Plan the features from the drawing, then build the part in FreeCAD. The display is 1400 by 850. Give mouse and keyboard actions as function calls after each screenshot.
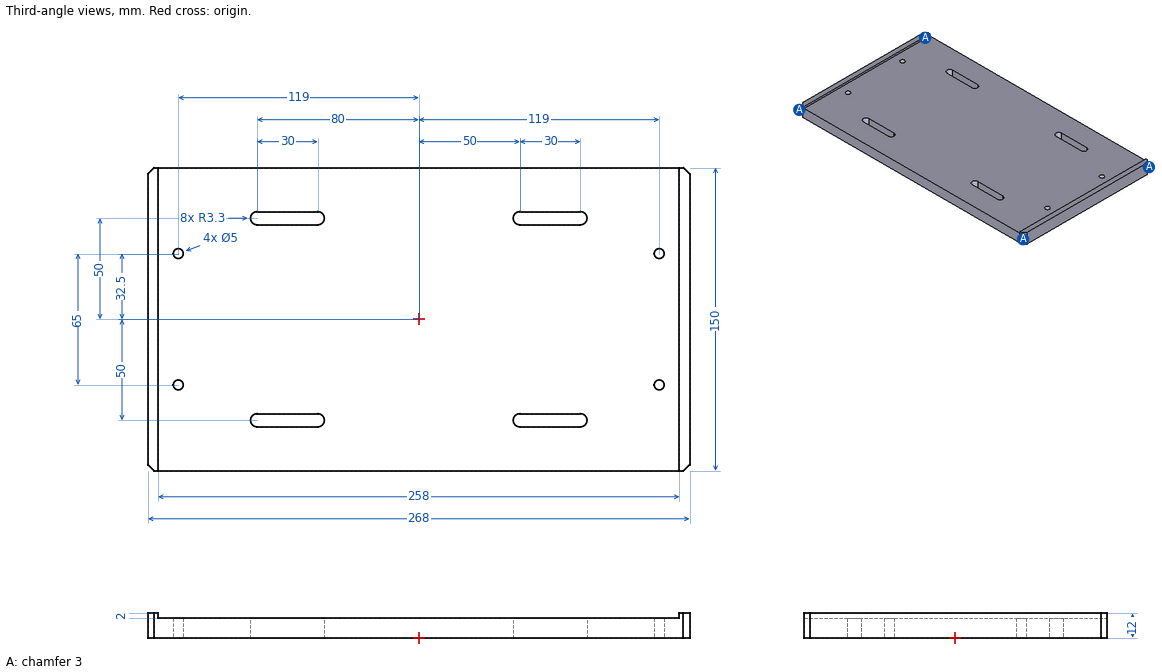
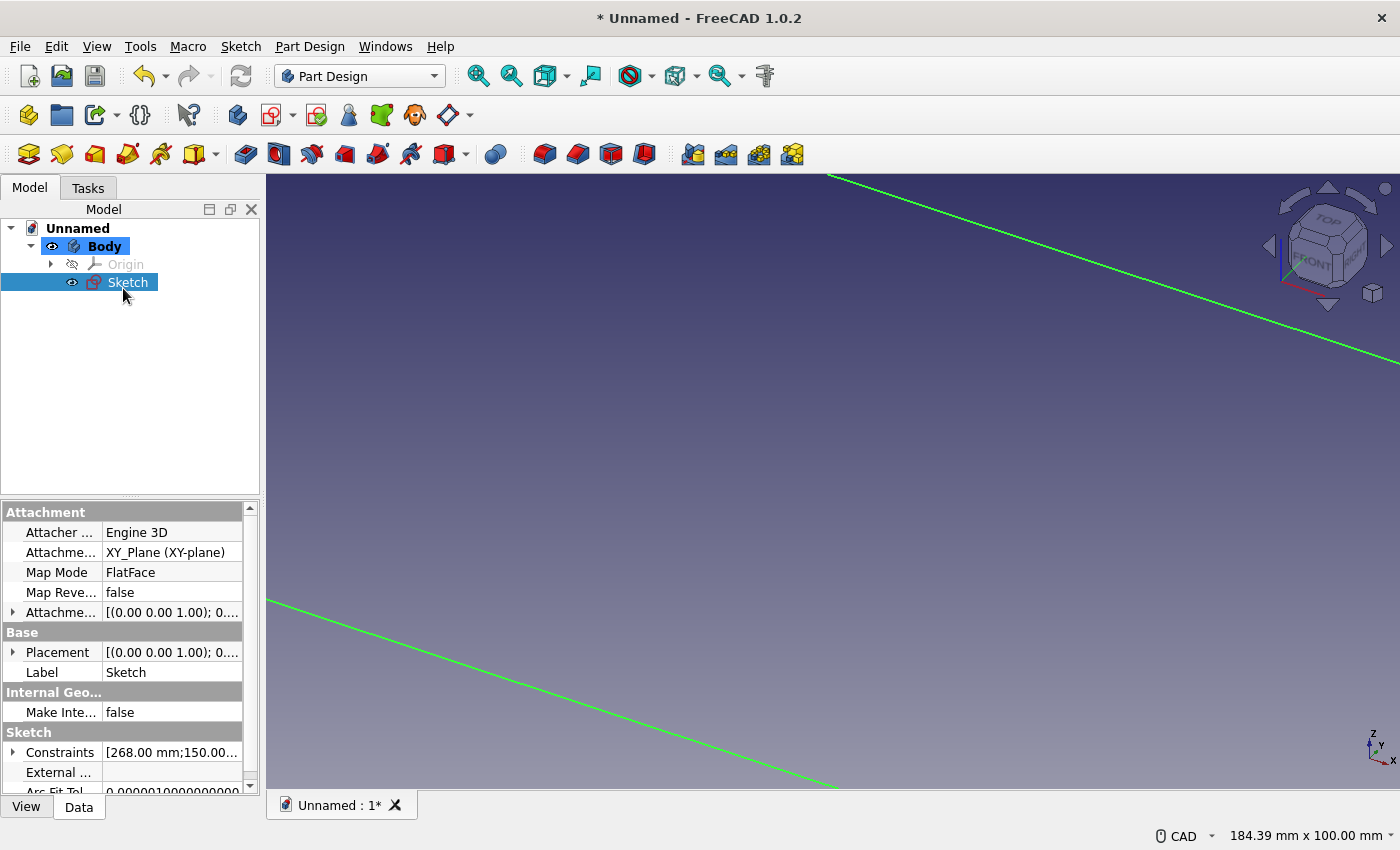
click(29, 154)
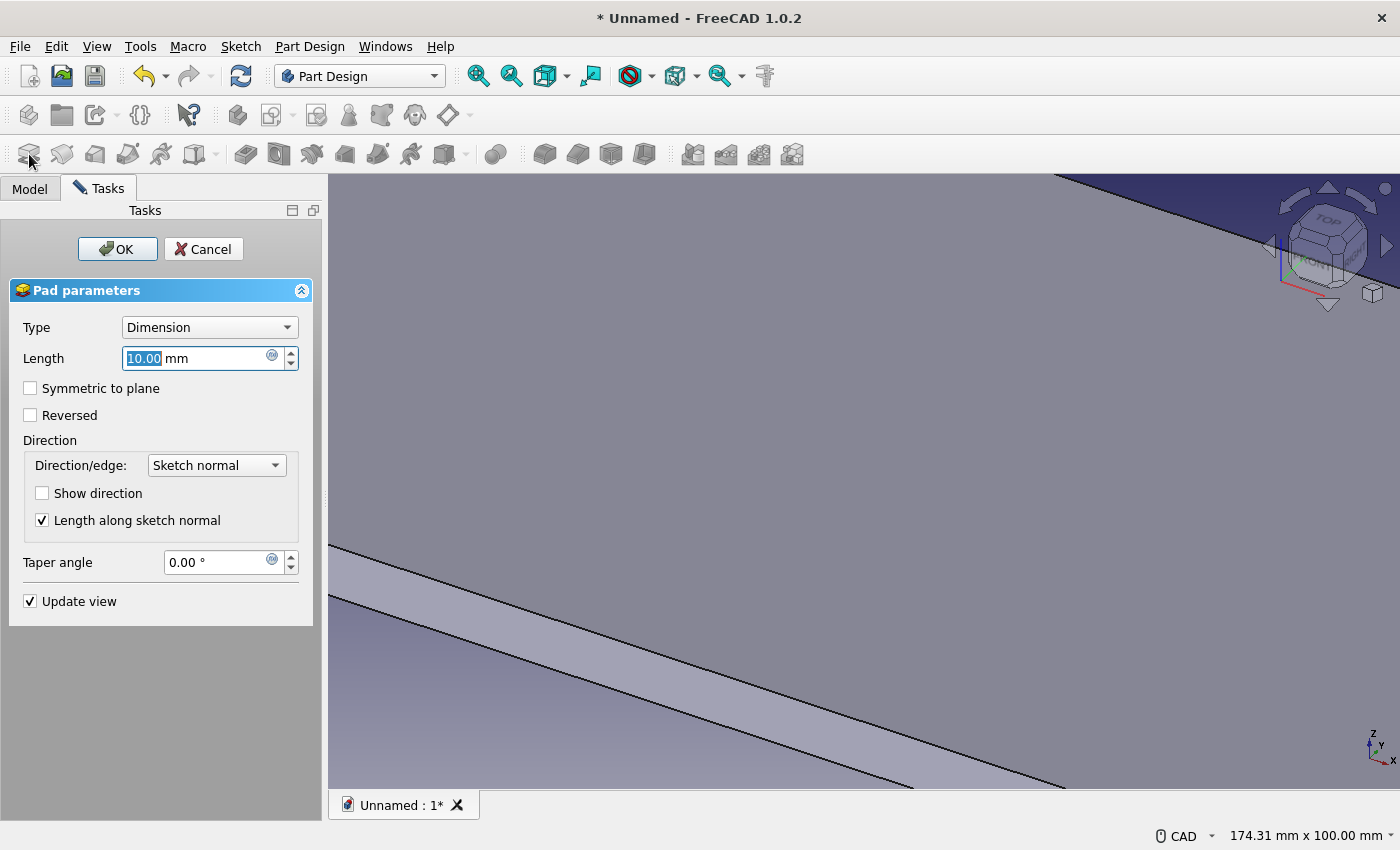
text(12)
key(Tab)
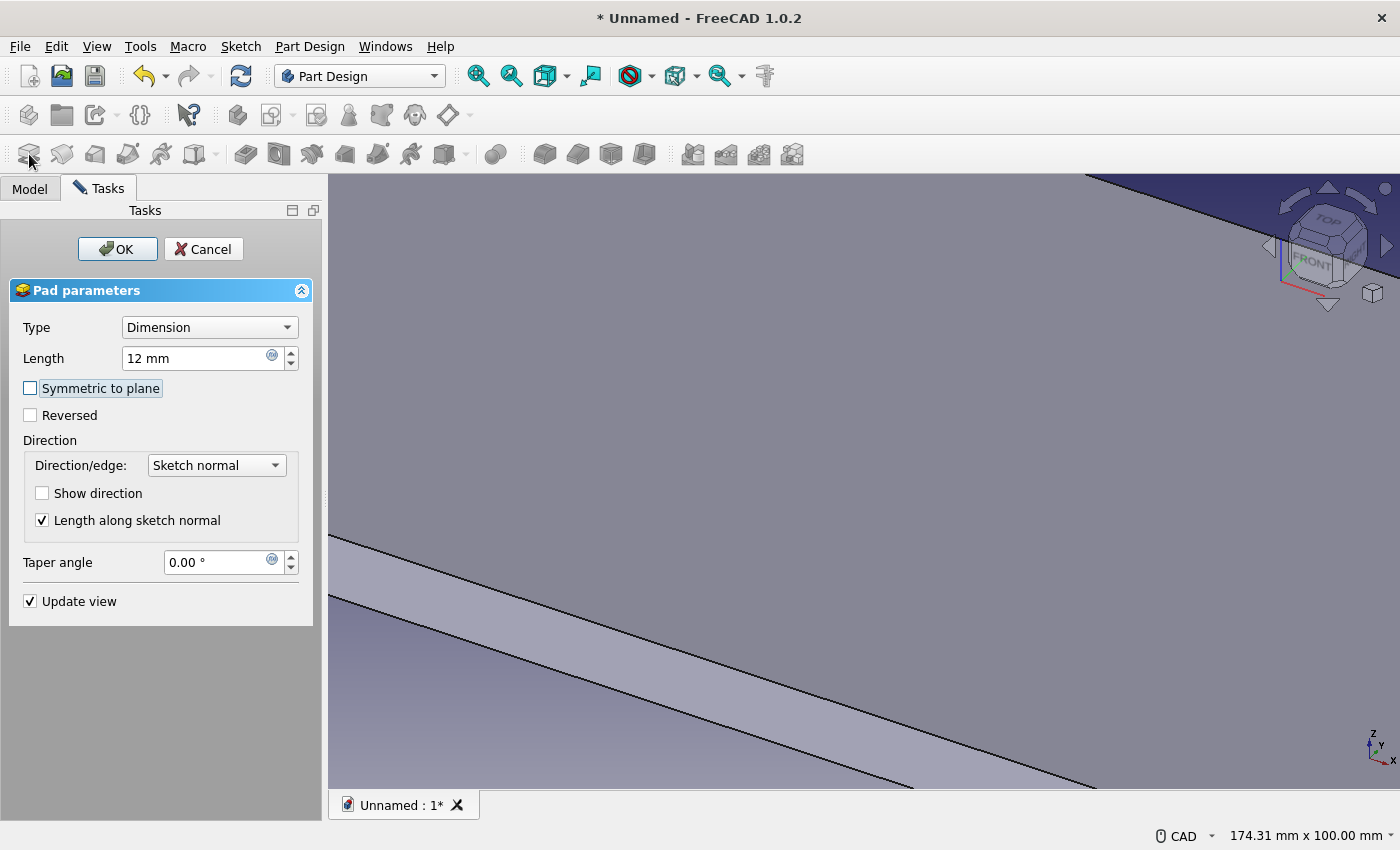
click(118, 249)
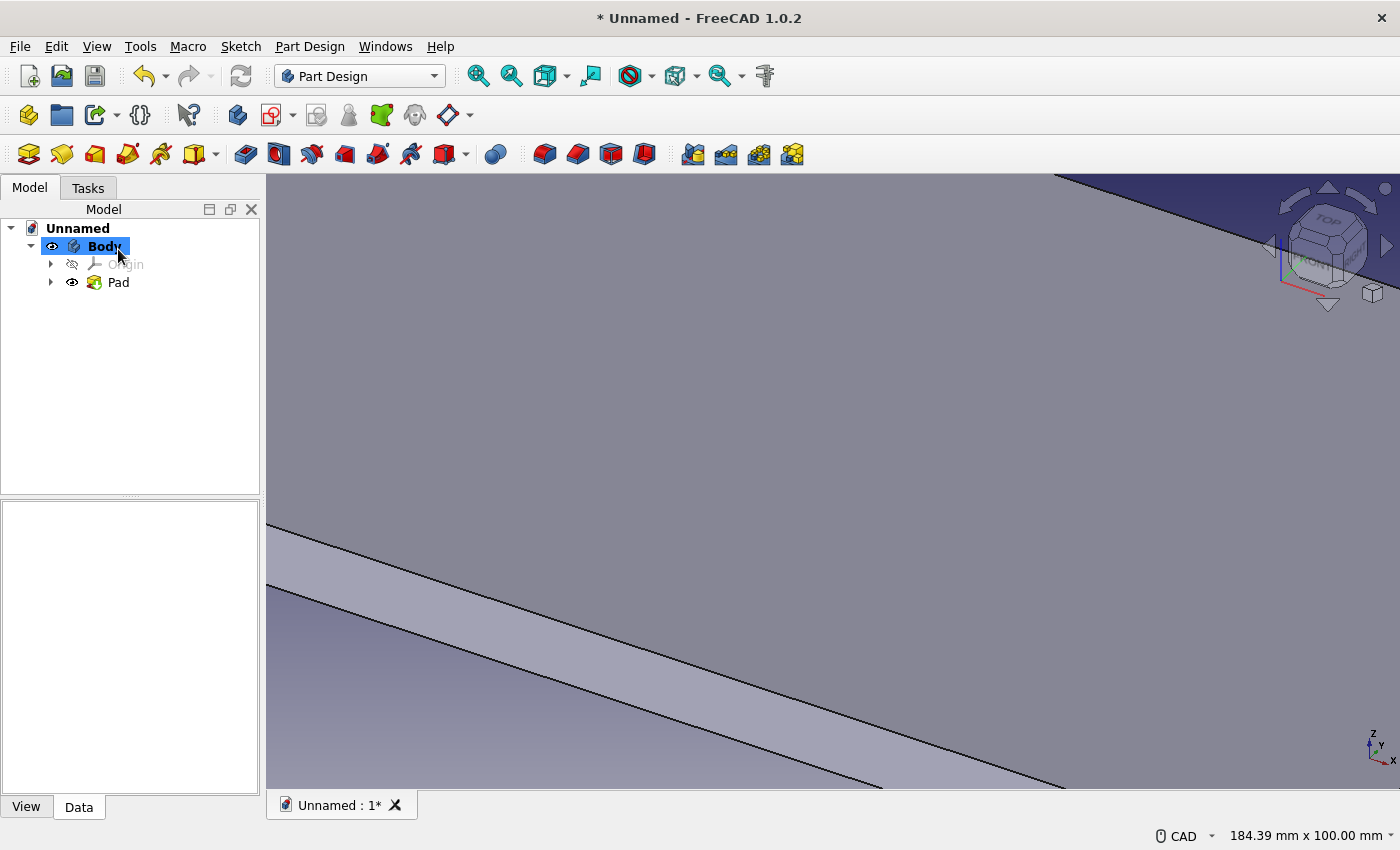
click(479, 76)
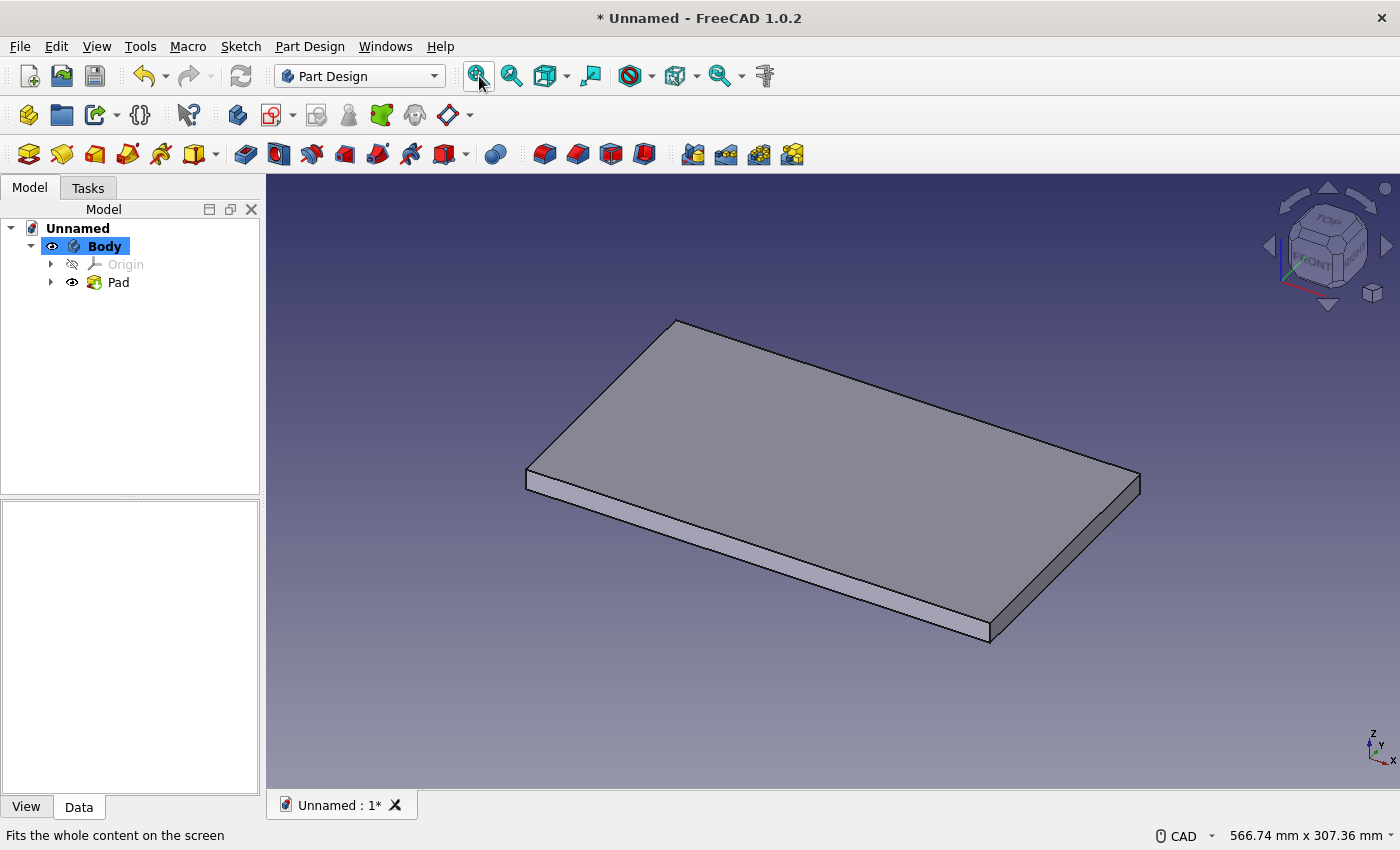
click(899, 493)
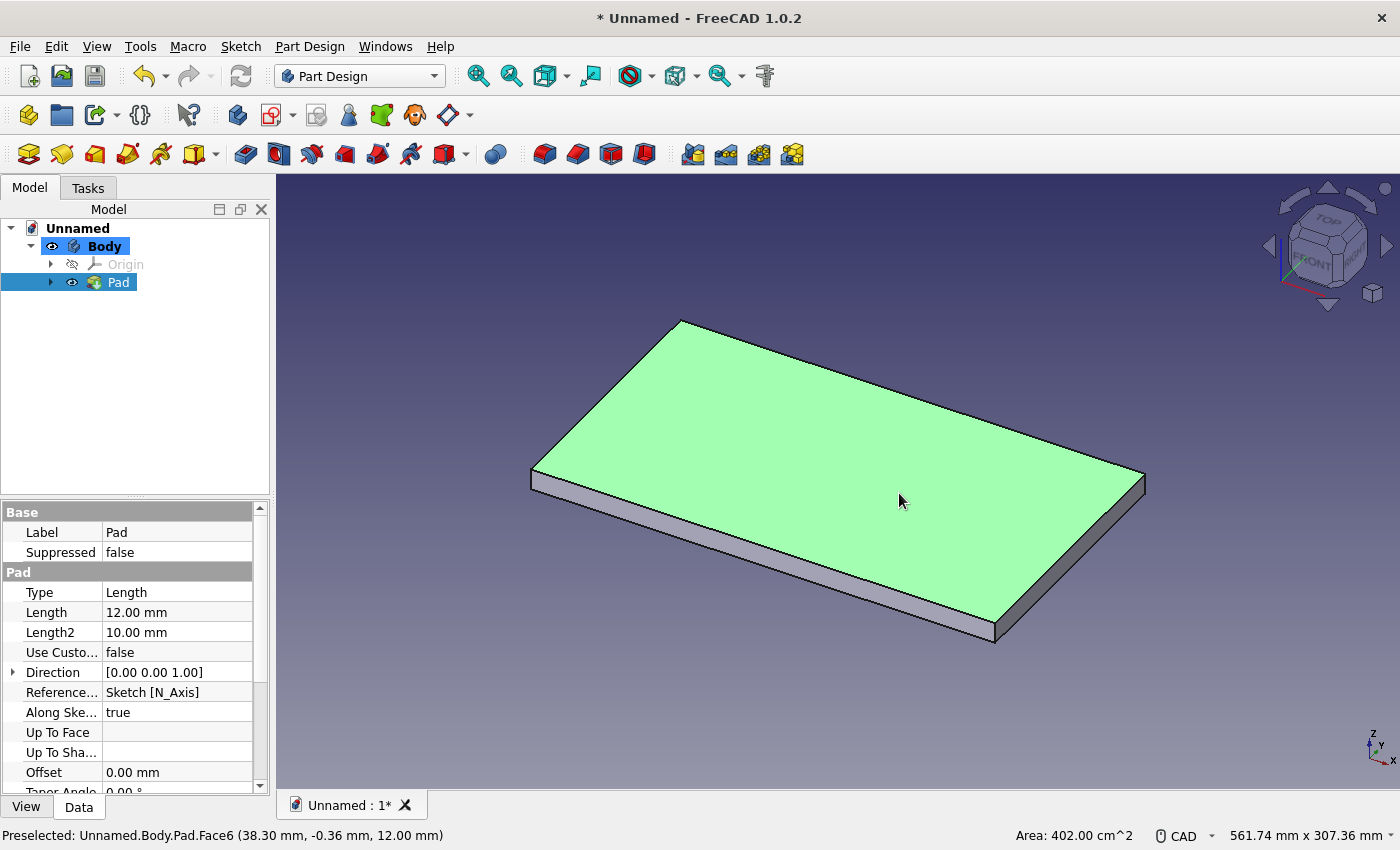
click(270, 116)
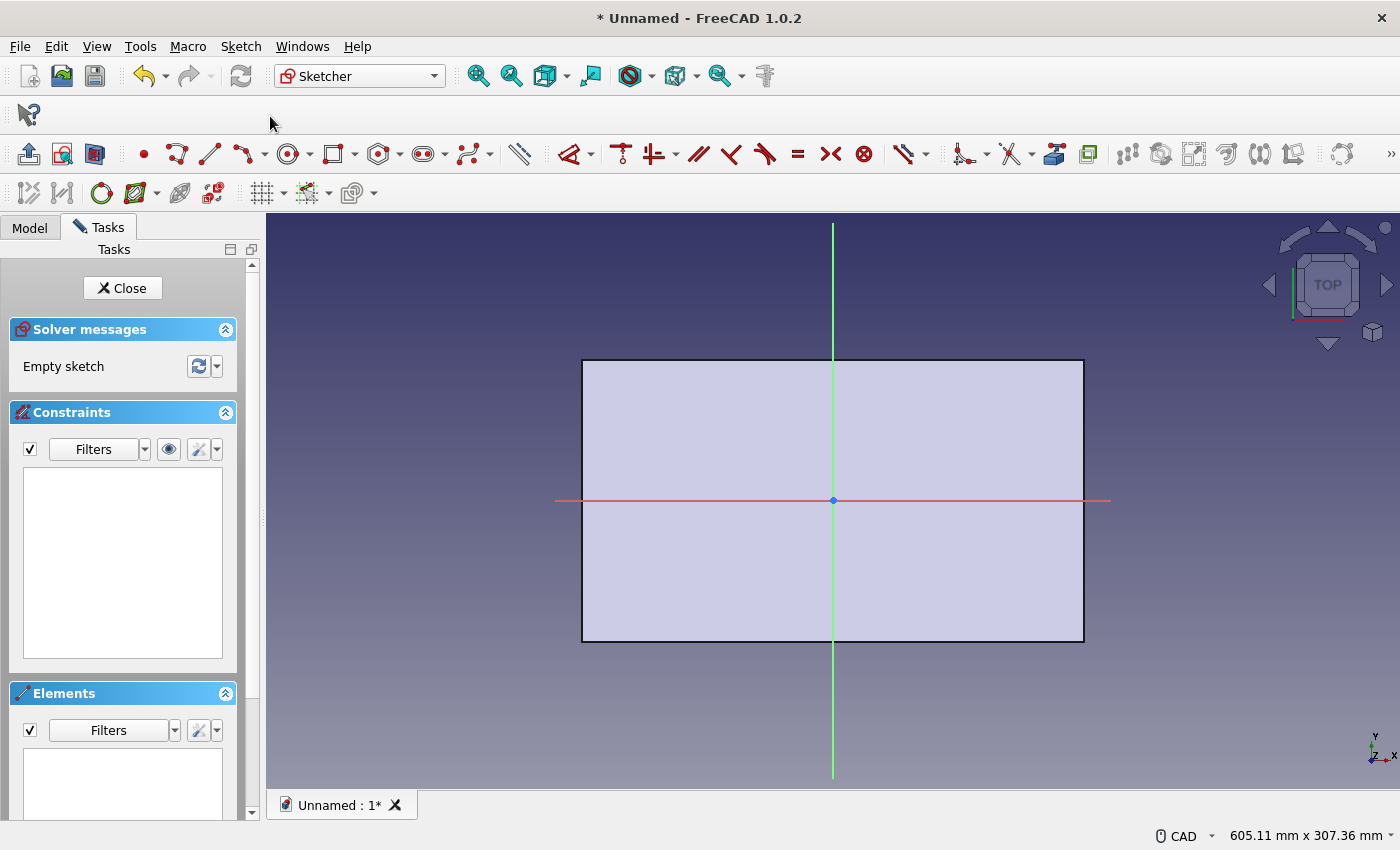
key(g)
key(v)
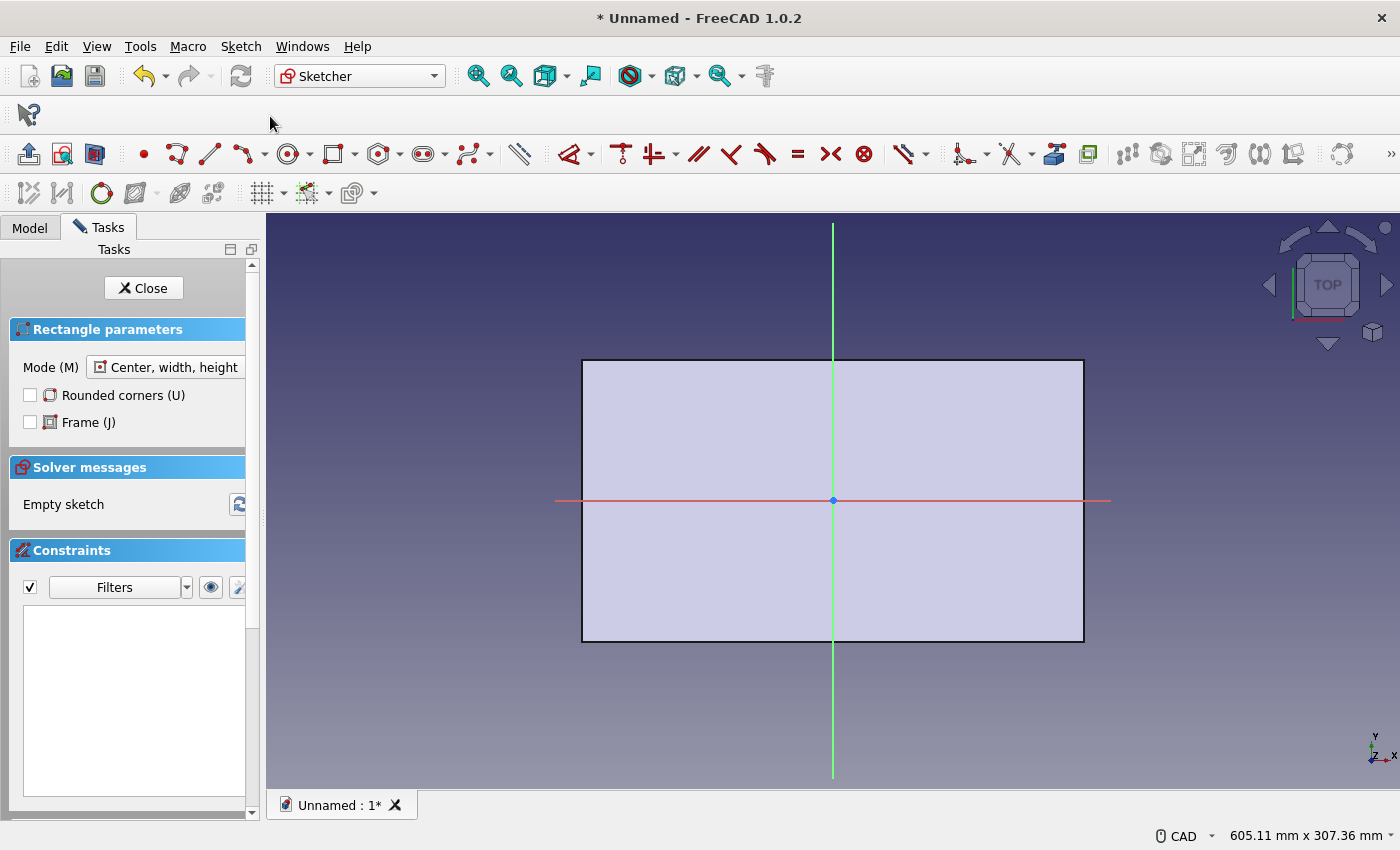
click(833, 501)
move(1075, 360)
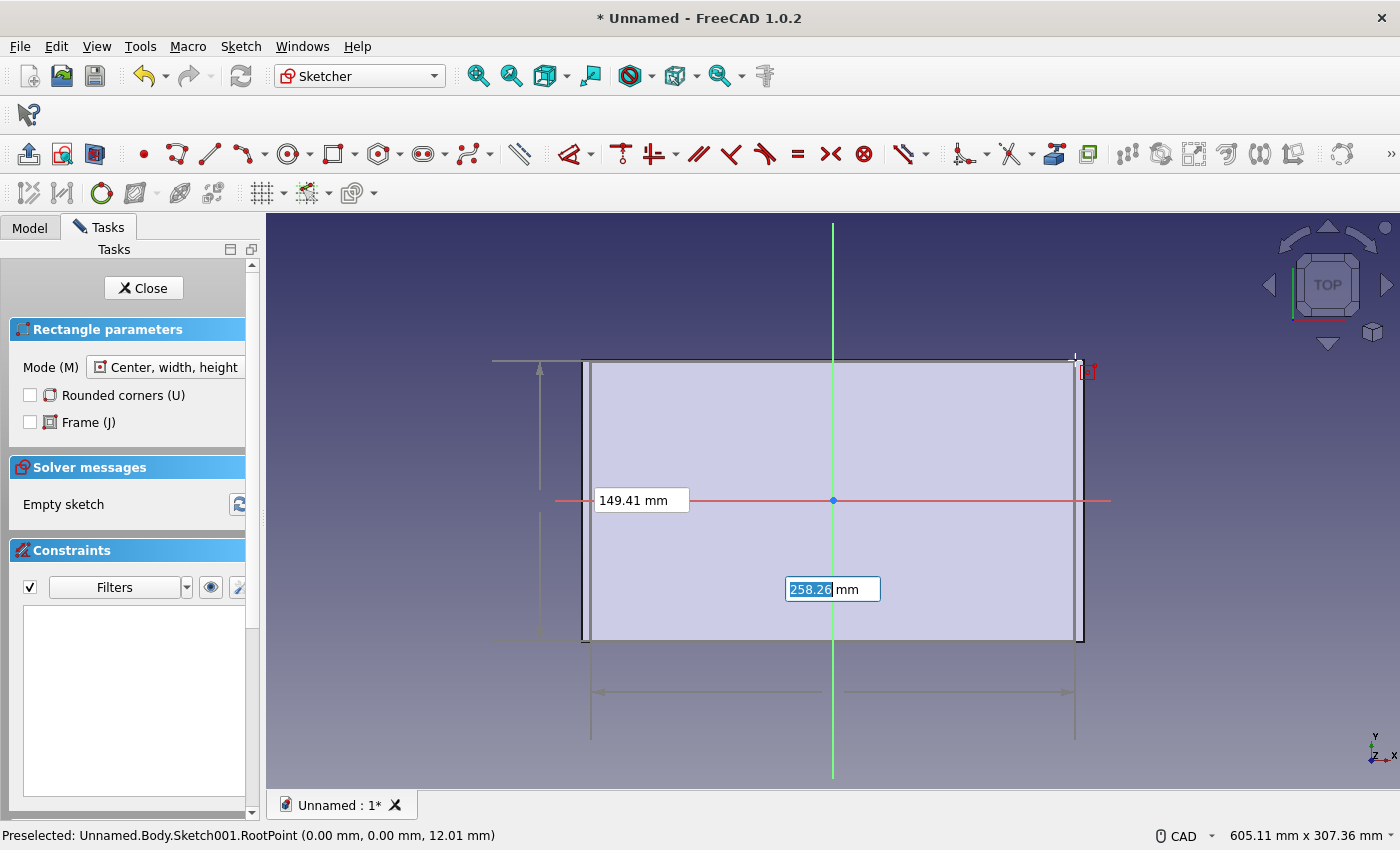
text(258)
key(Tab)
text(150)
key(Return)
key(Escape)